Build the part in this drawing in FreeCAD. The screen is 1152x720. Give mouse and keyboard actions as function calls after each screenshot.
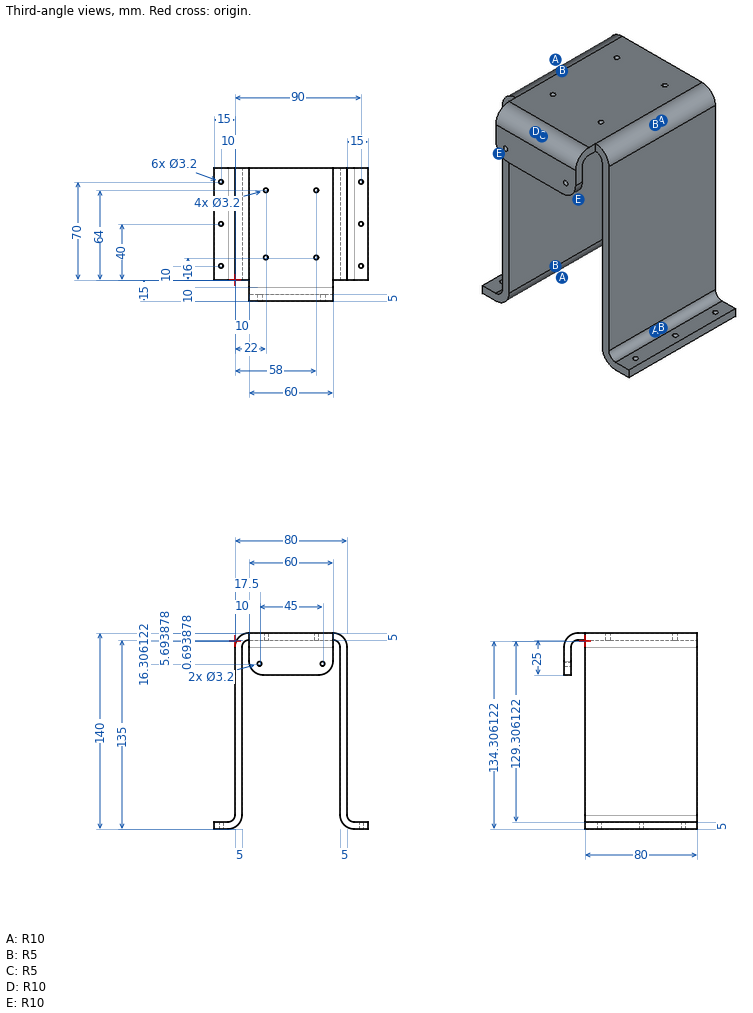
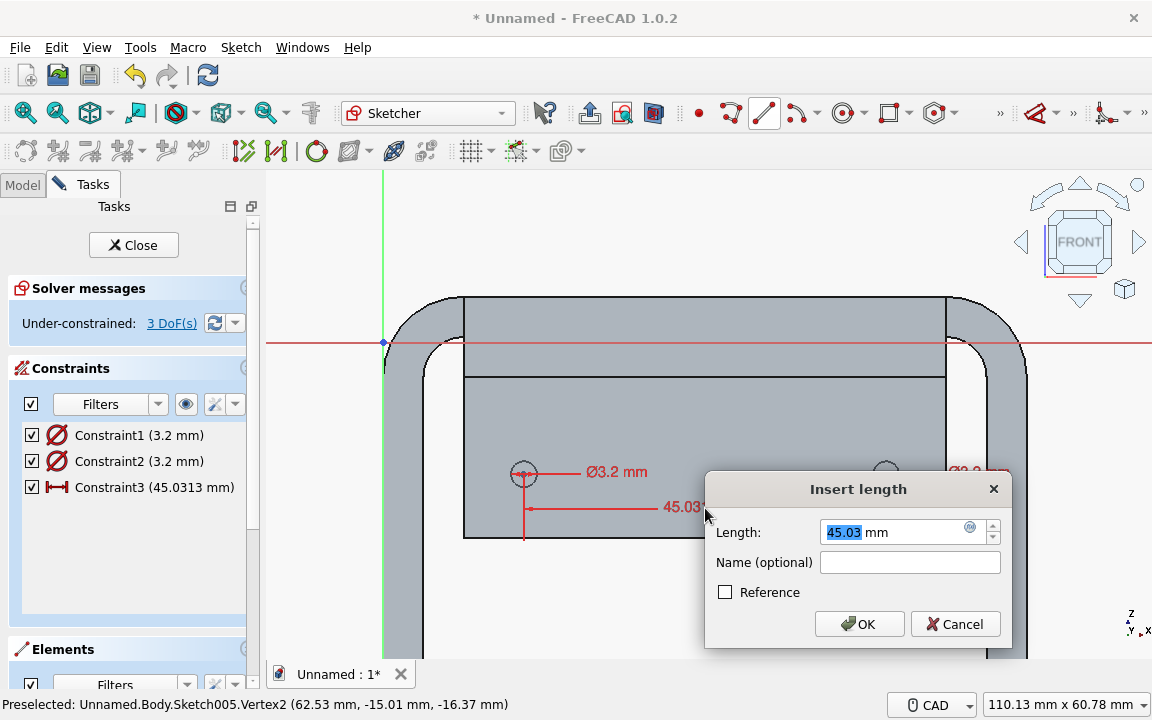
text(45)
key(Return)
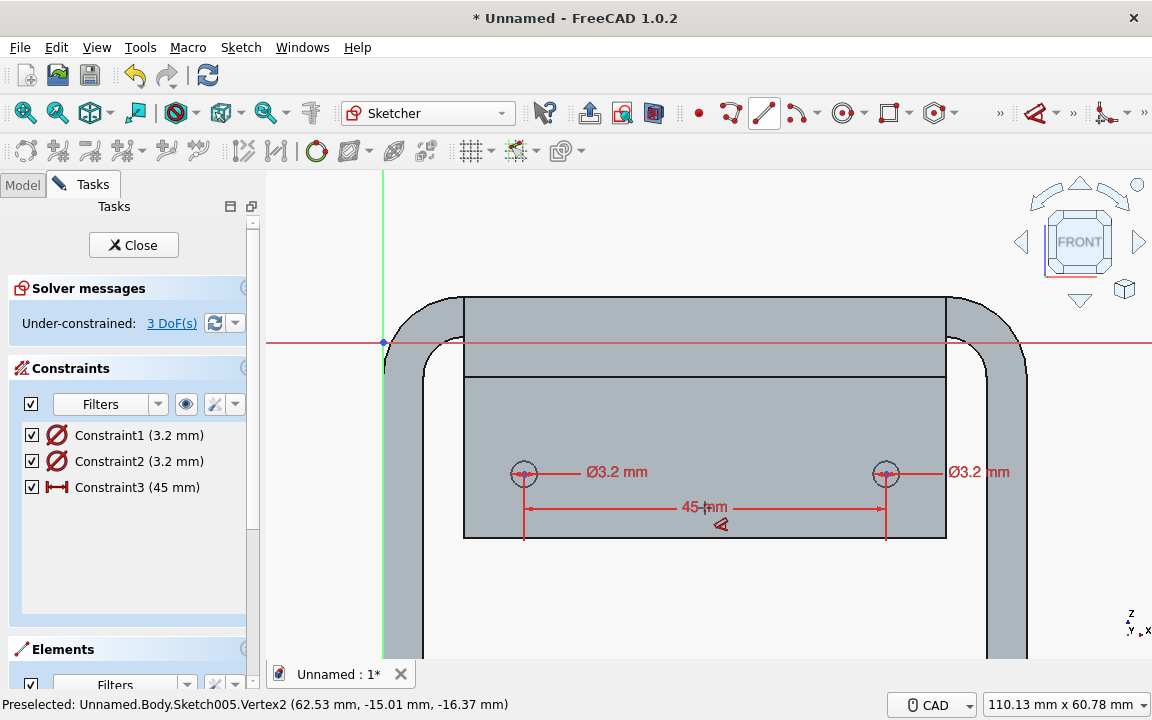
click(524, 474)
click(454, 309)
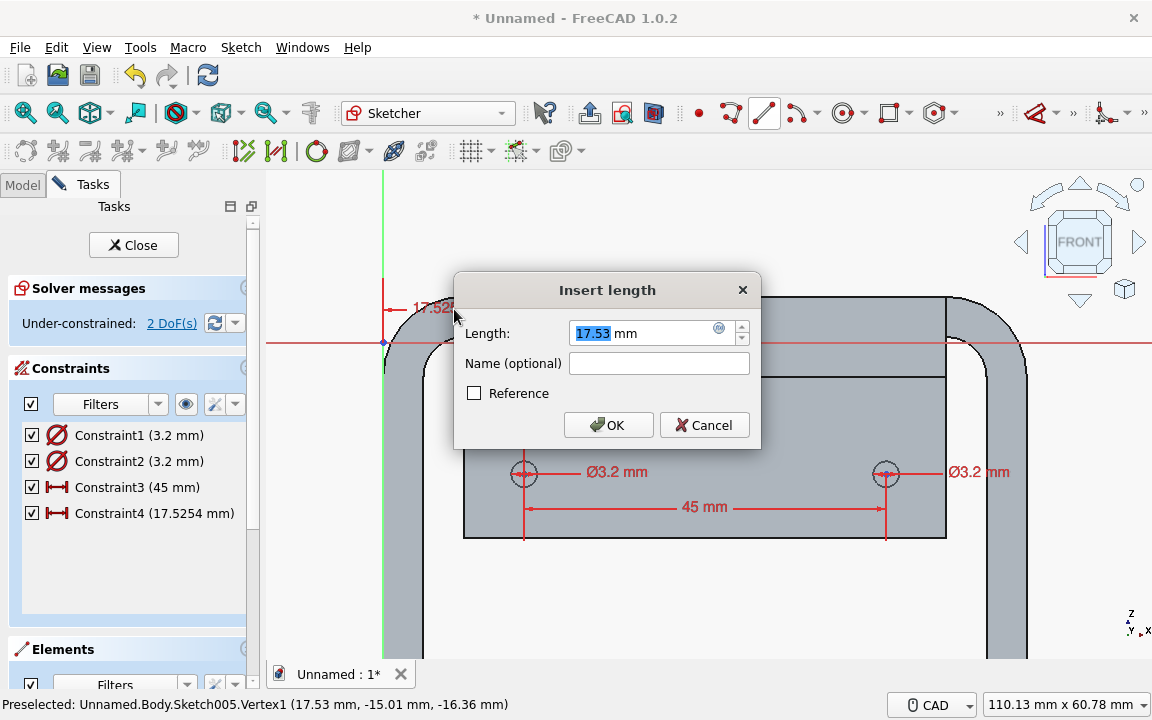
text(17.5)
key(Return)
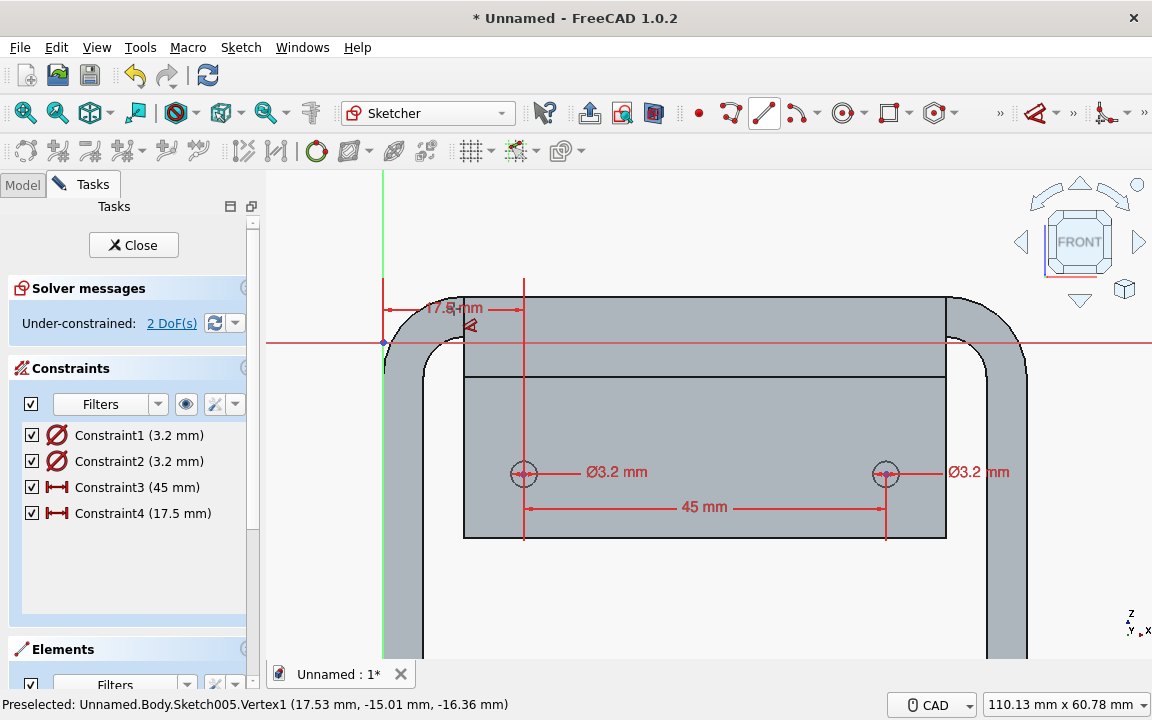
click(524, 474)
click(349, 408)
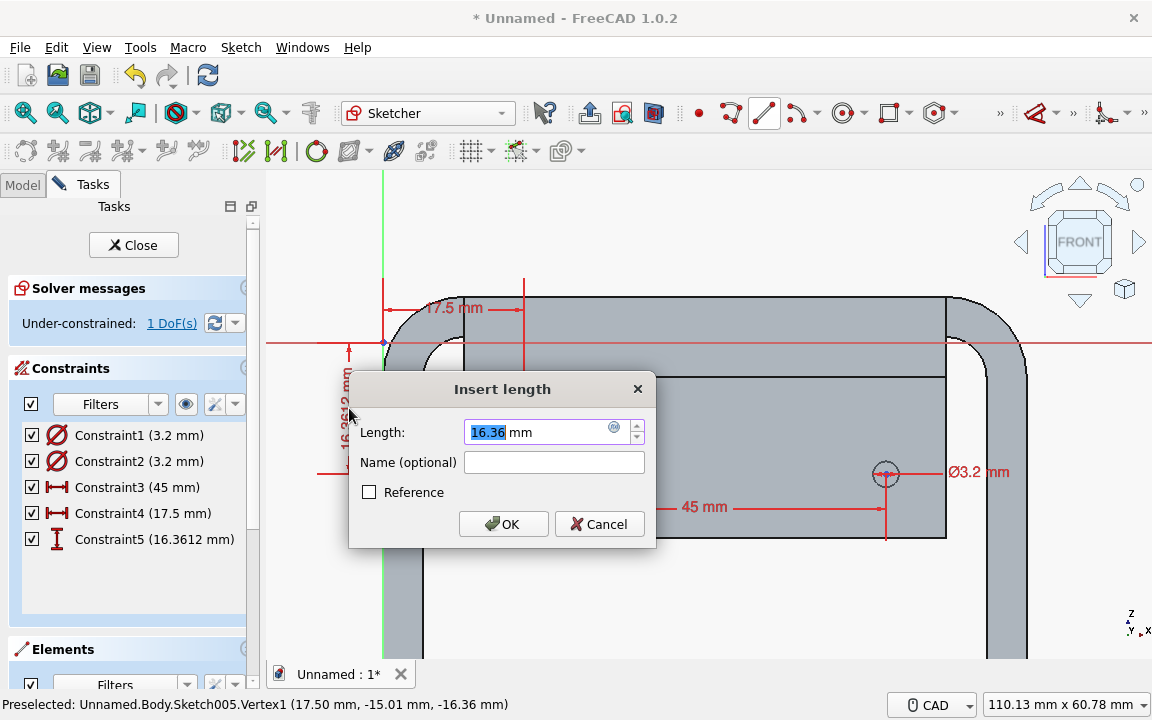
text(16.306122)
key(Return)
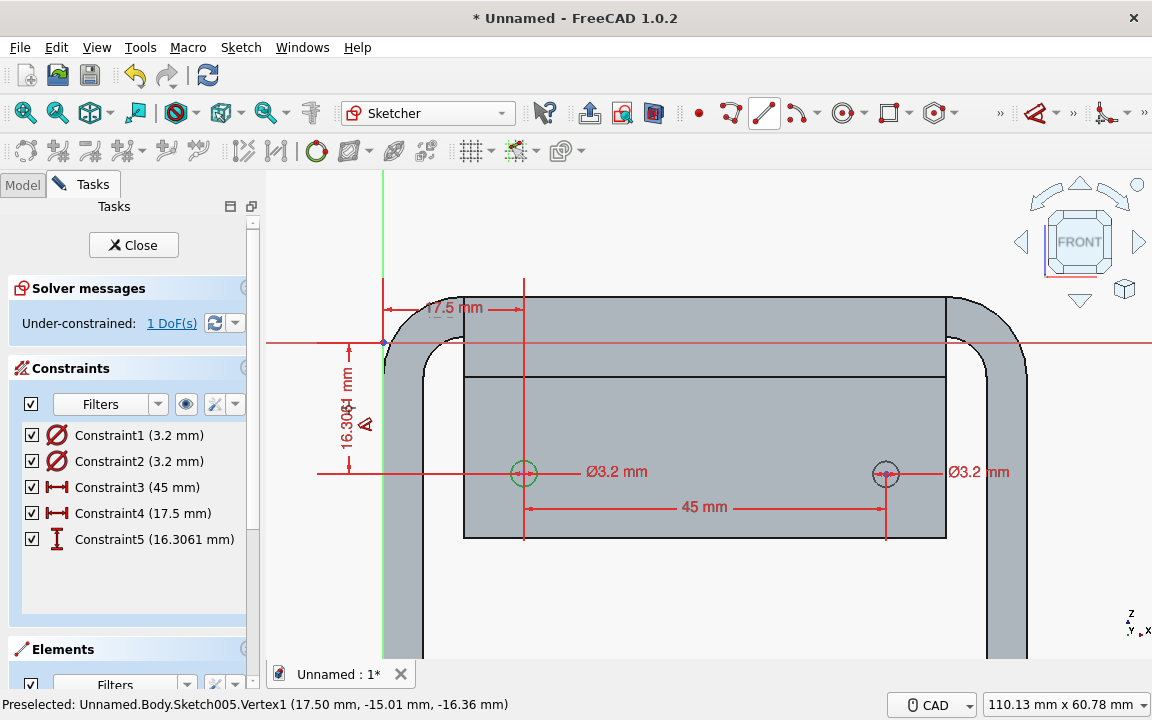
click(886, 474)
click(349, 378)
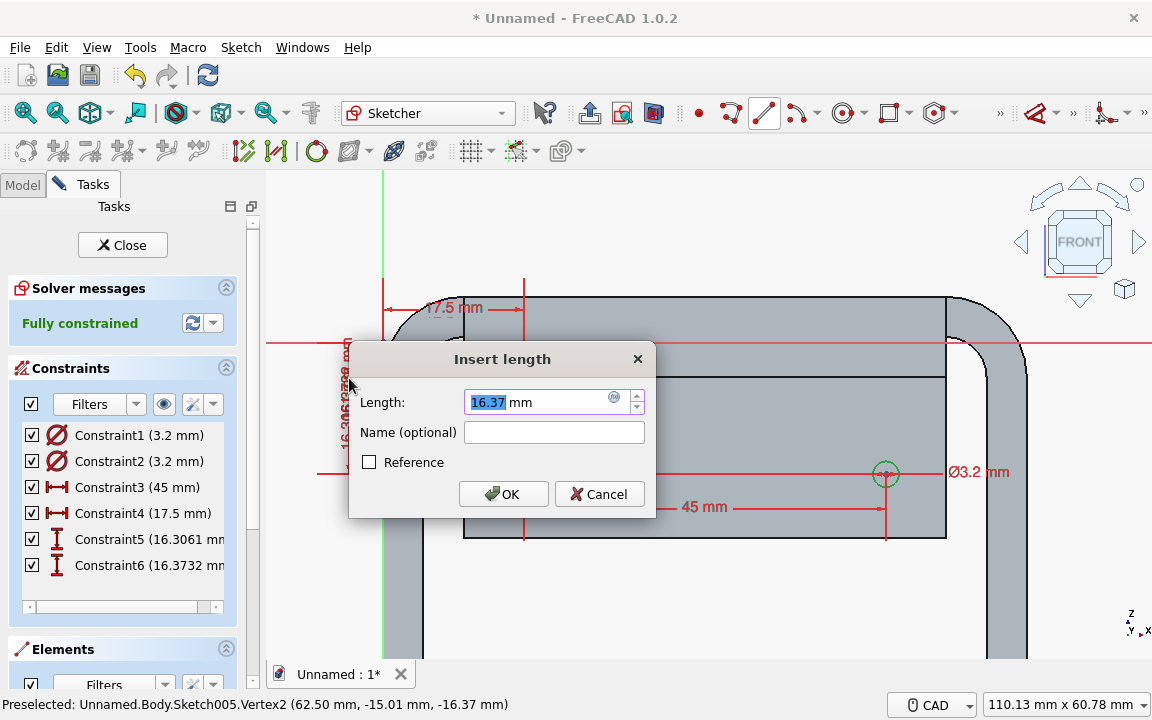
text(16.306122)
key(Return)
key(Escape)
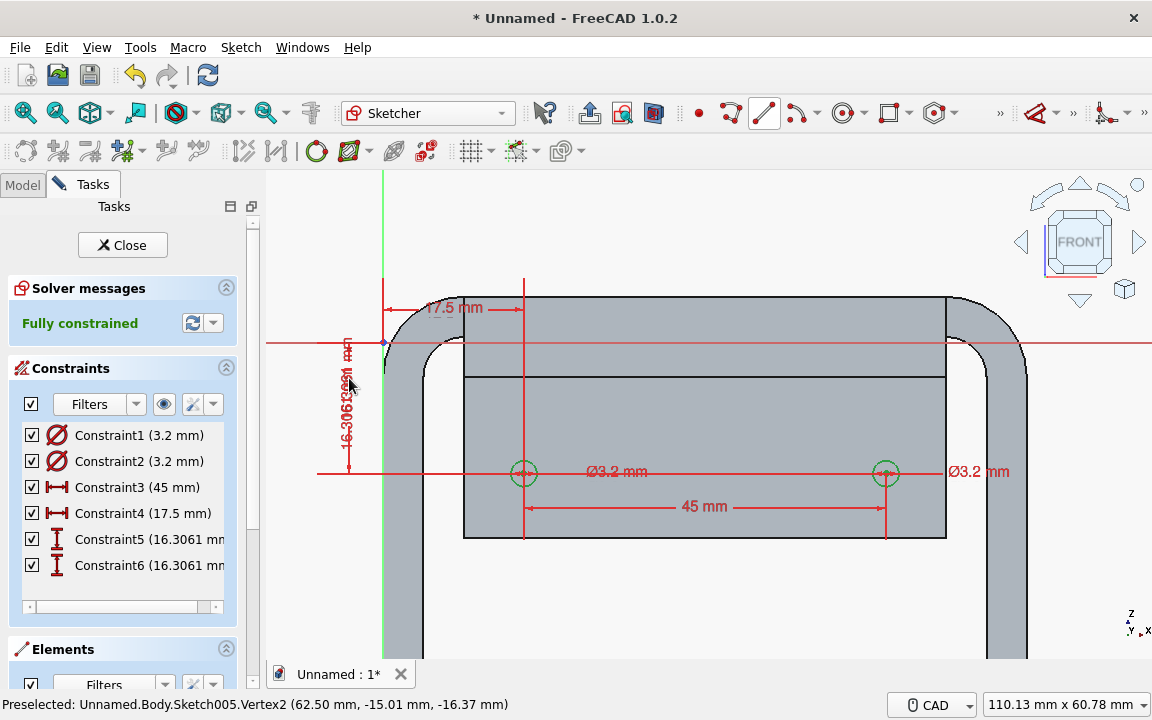
click(123, 245)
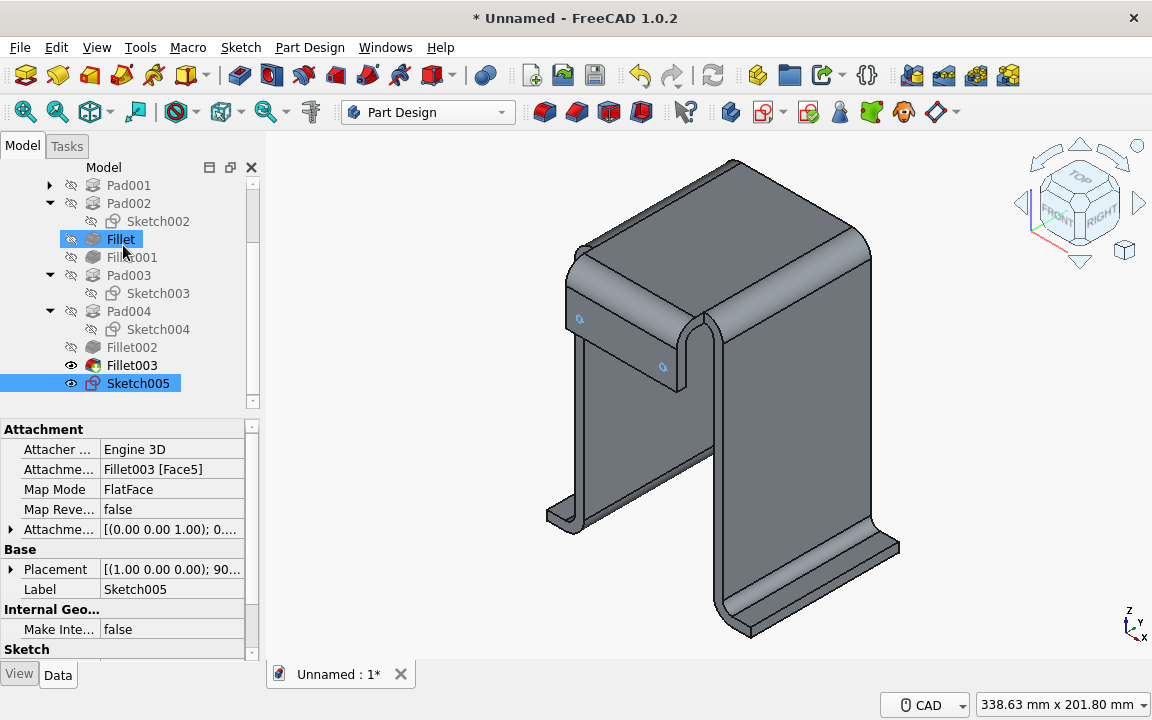
click(240, 76)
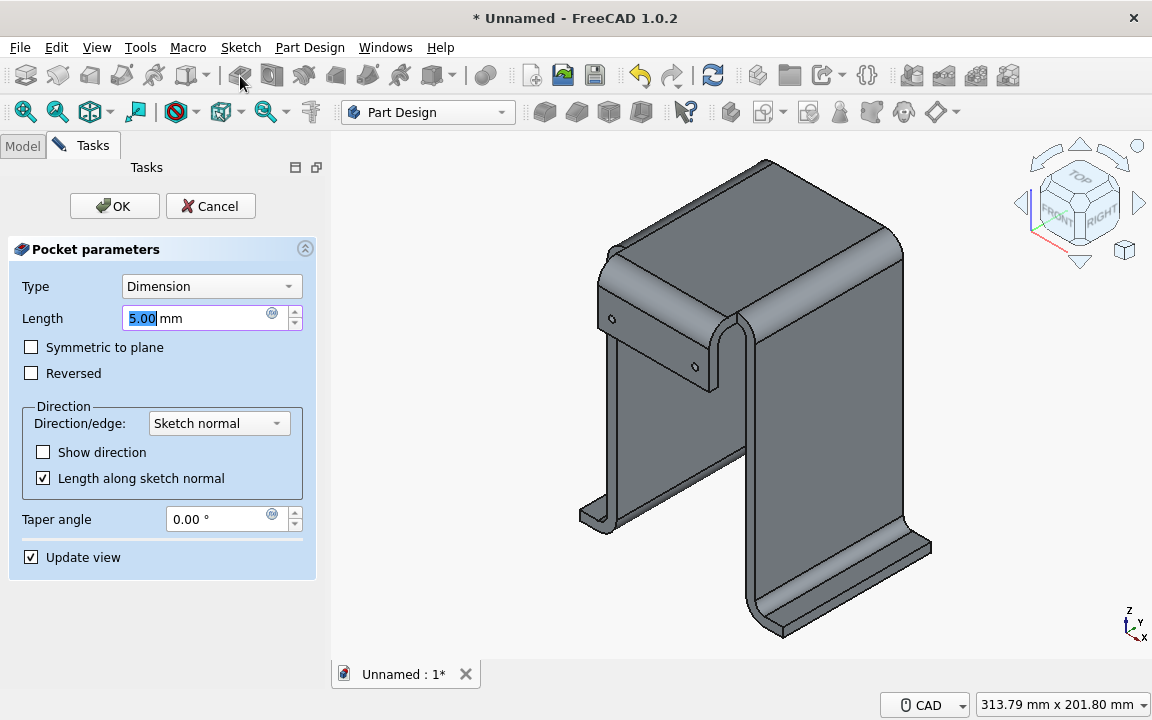
text(10)
key(Tab)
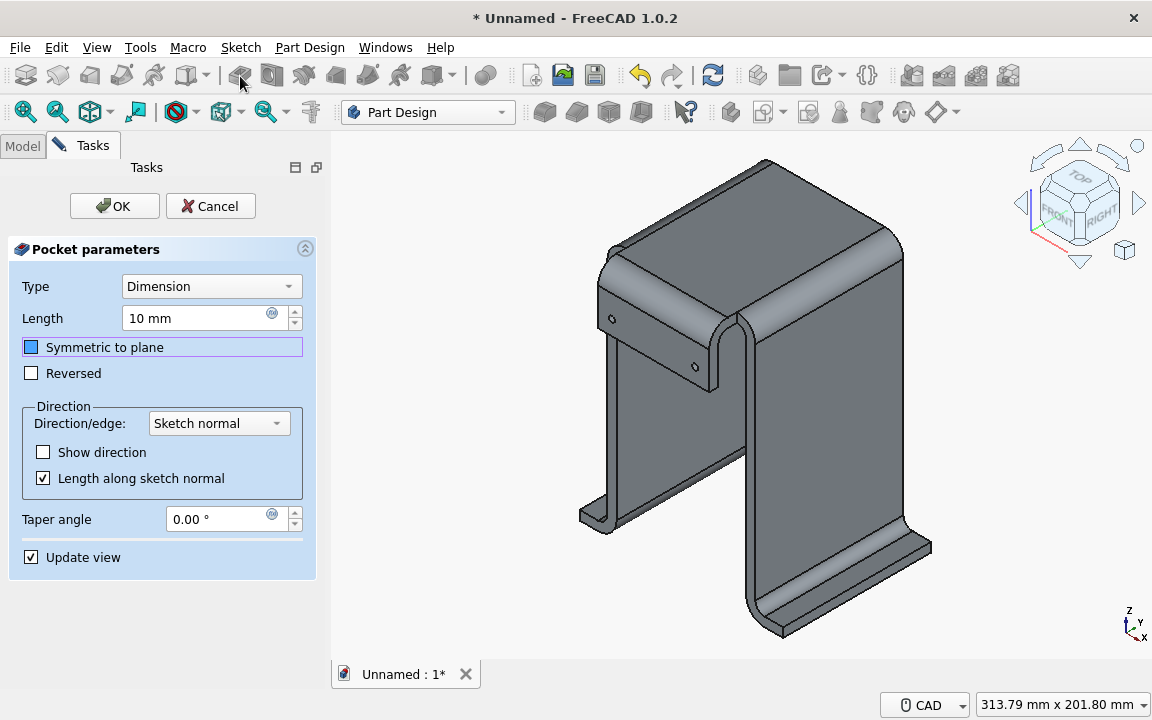
click(115, 206)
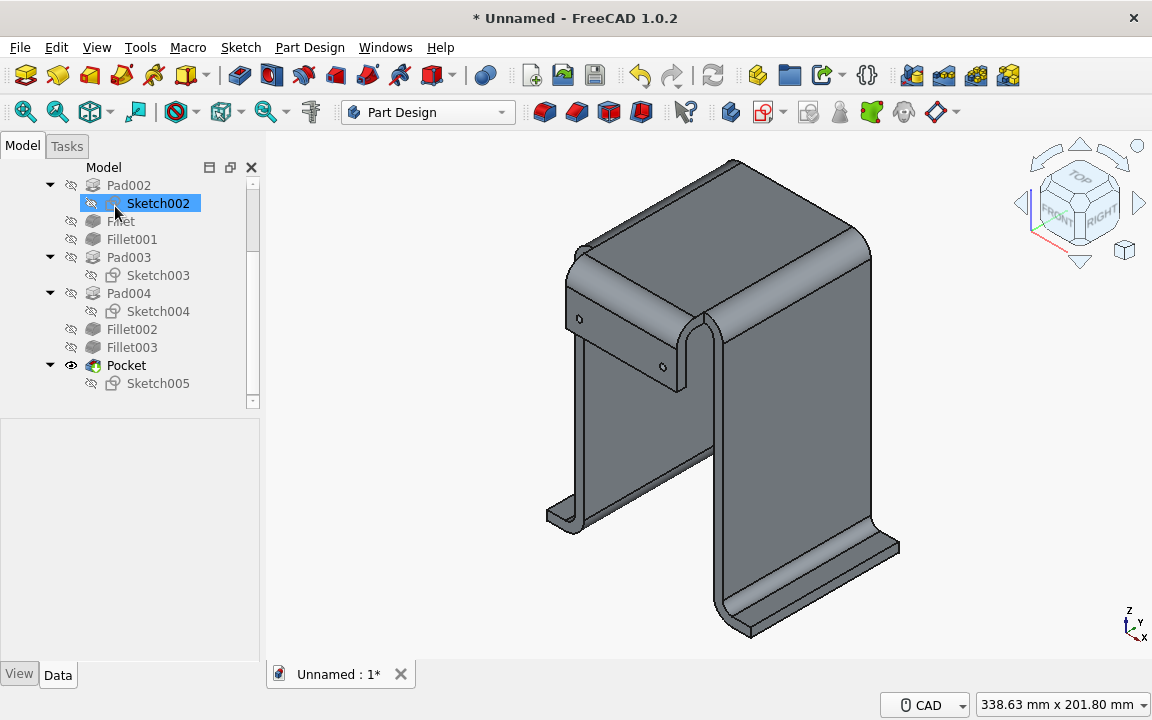
scroll(681, 389, up, 6)